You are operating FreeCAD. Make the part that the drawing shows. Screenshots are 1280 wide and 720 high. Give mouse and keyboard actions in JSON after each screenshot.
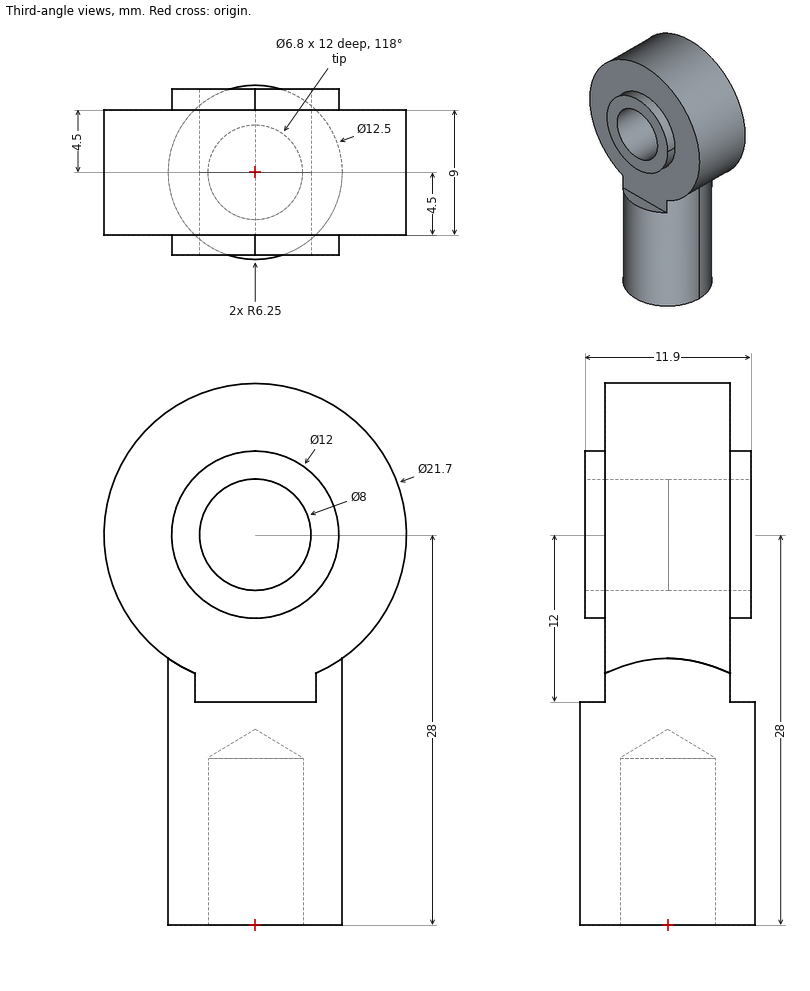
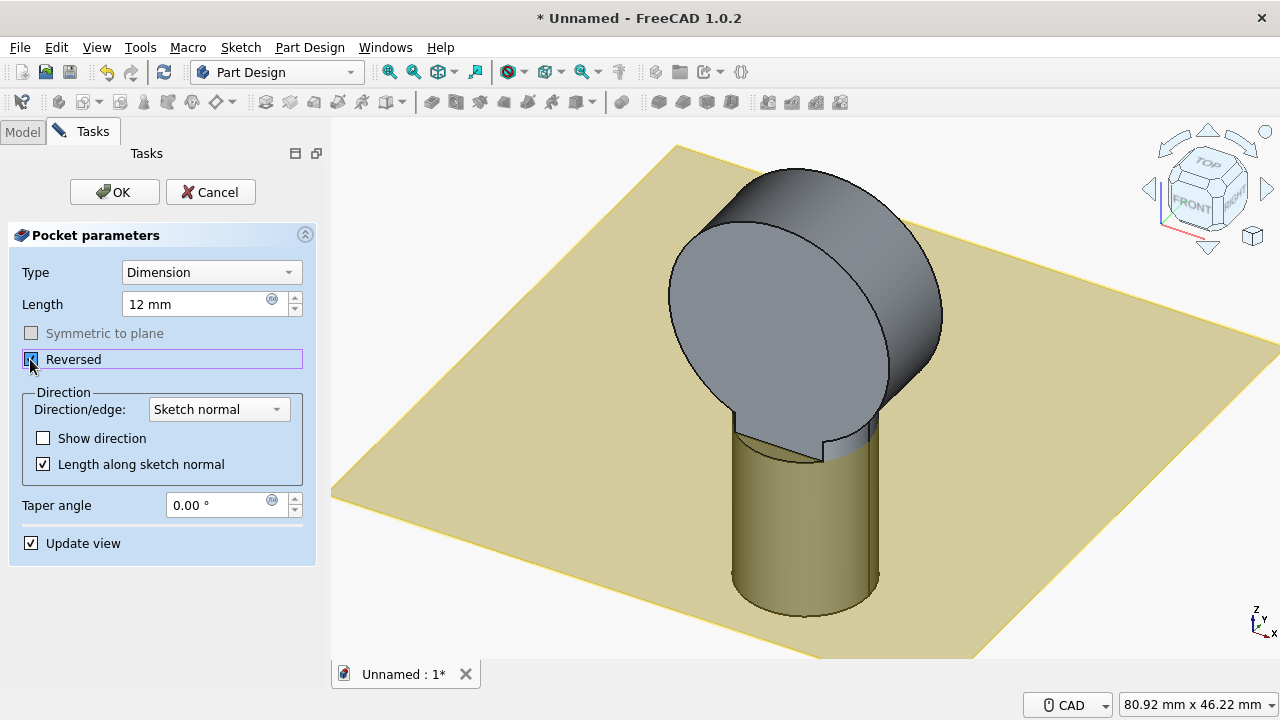
{"action": "left_click", "coordinate": [115, 192]}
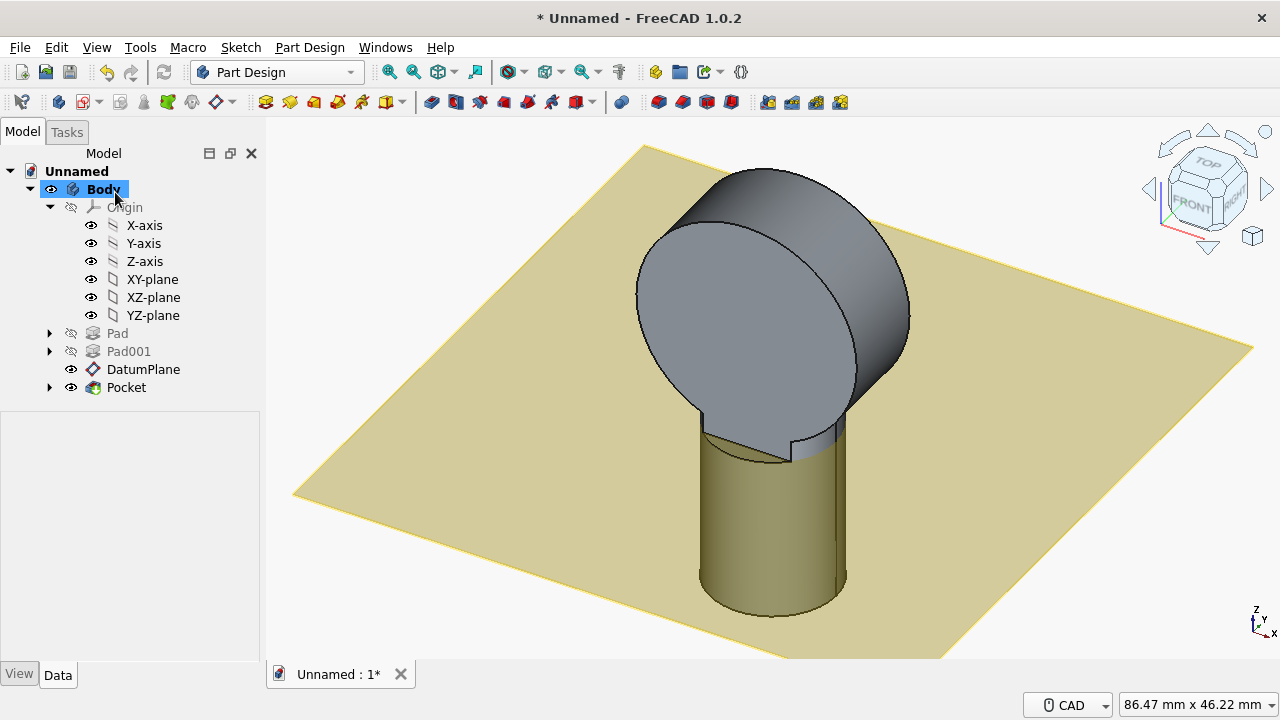
{"action": "left_click", "coordinate": [116, 369]}
{"action": "key", "text": "space"}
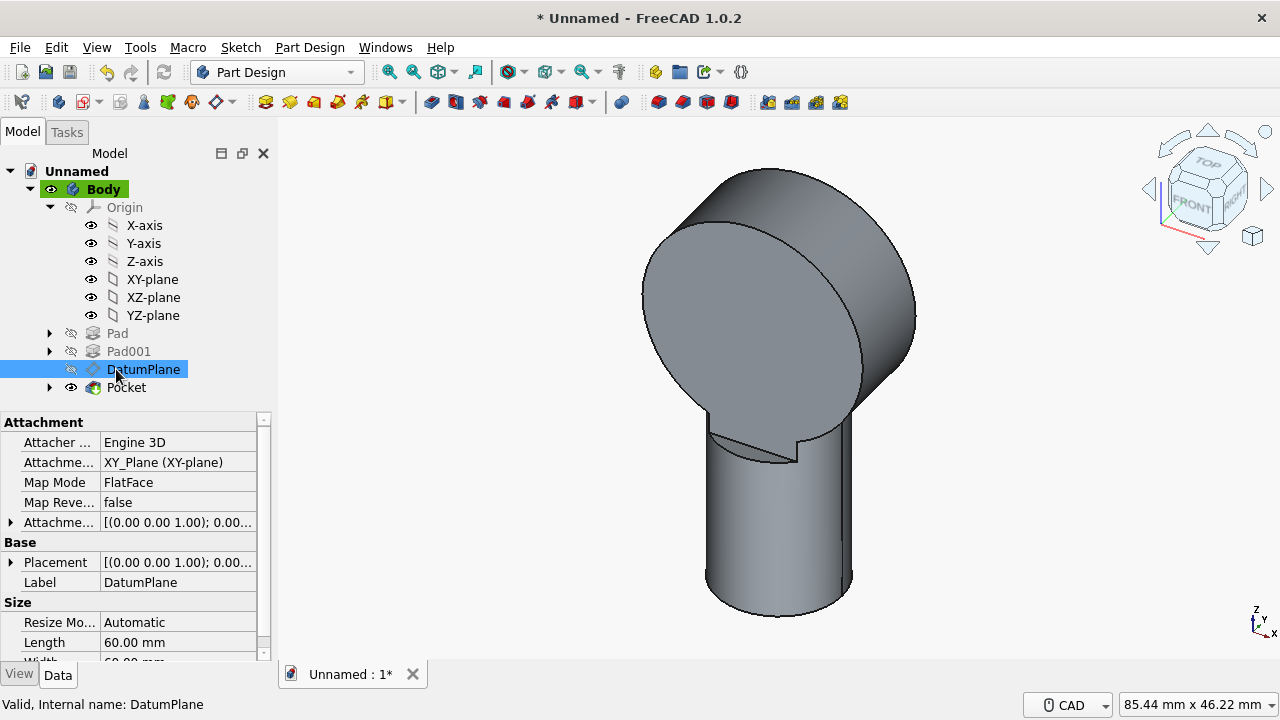
{"action": "left_click", "coordinate": [753, 336]}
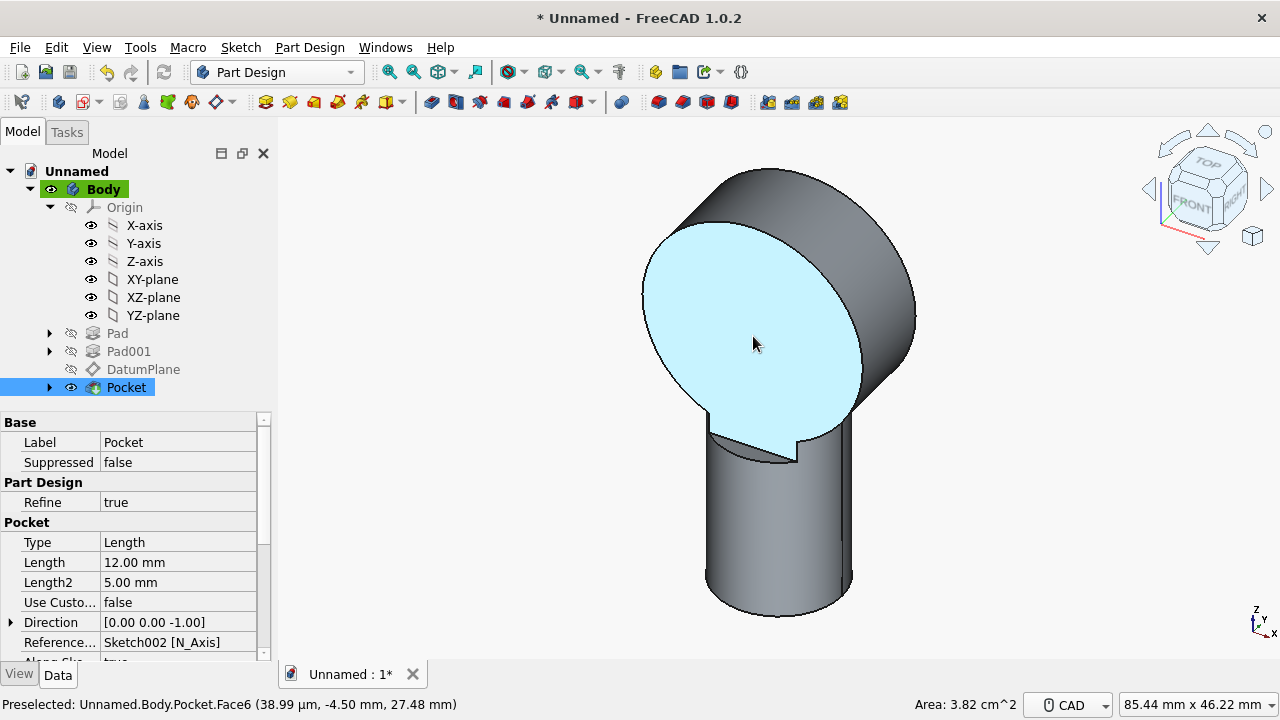
{"action": "left_click", "coordinate": [84, 102]}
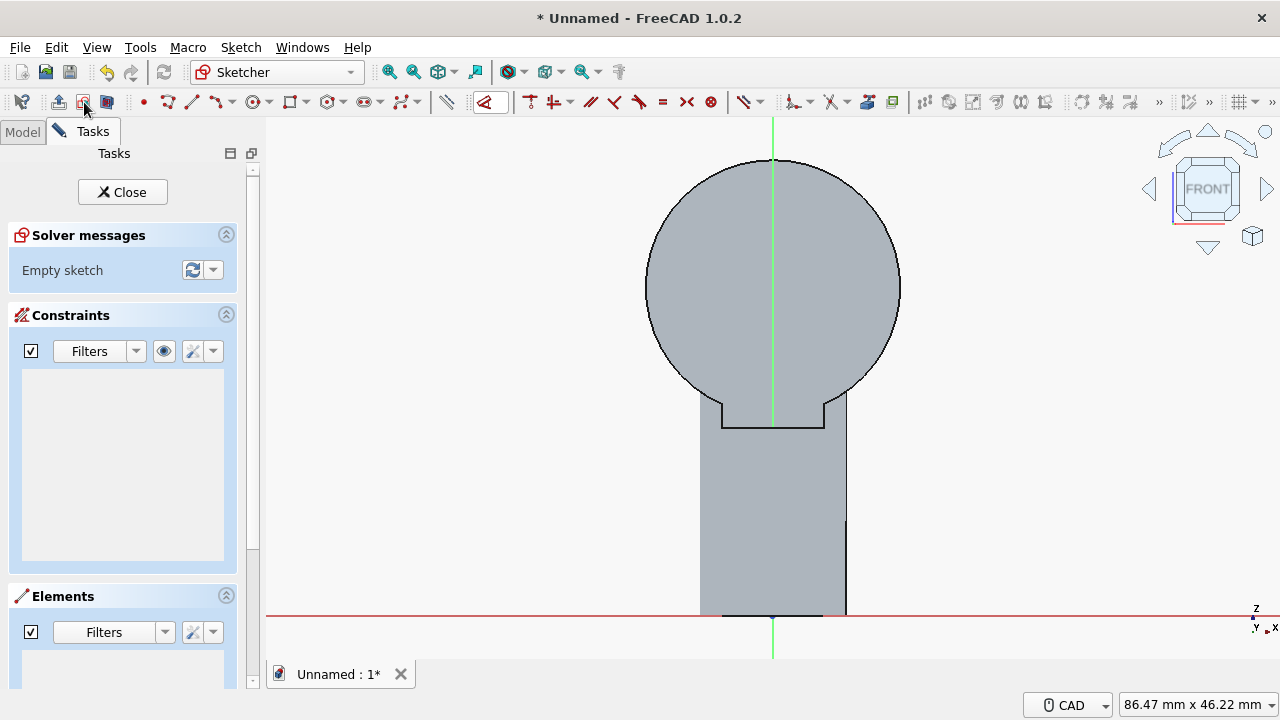
{"action": "key", "text": "q s"}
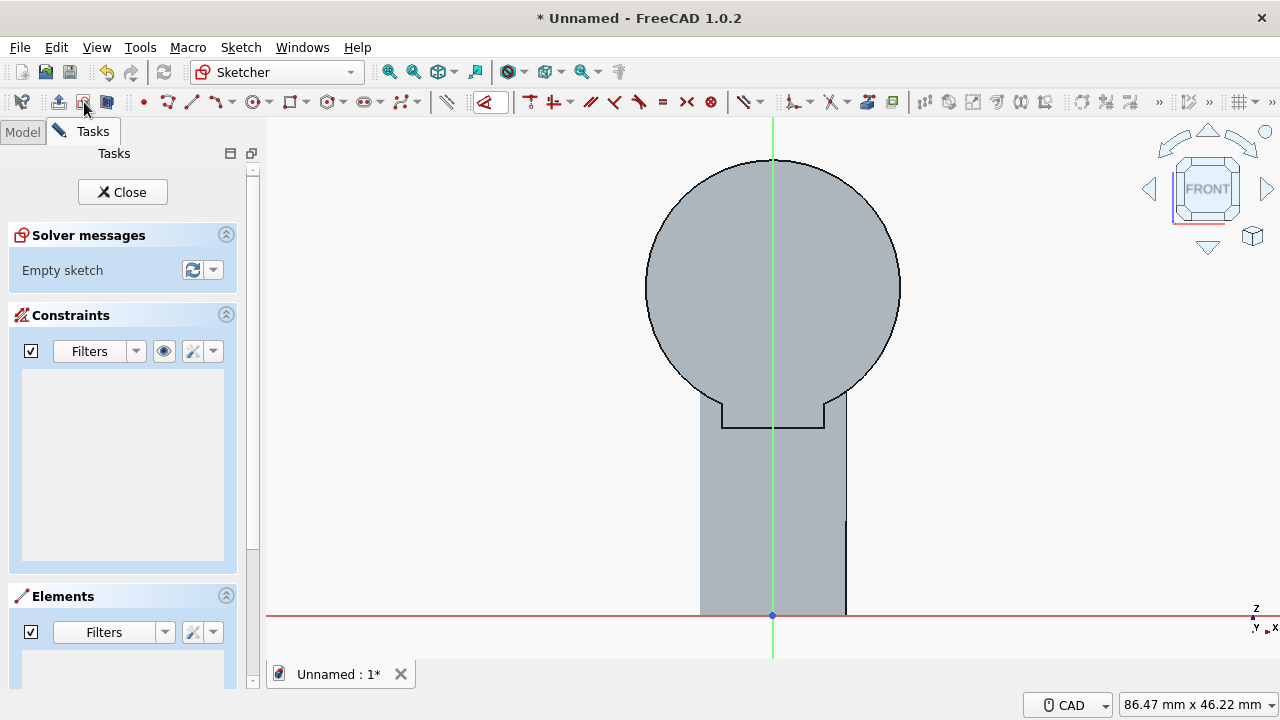
{"action": "scroll", "coordinate": [803, 244], "scroll_direction": "up", "scroll_amount": 6}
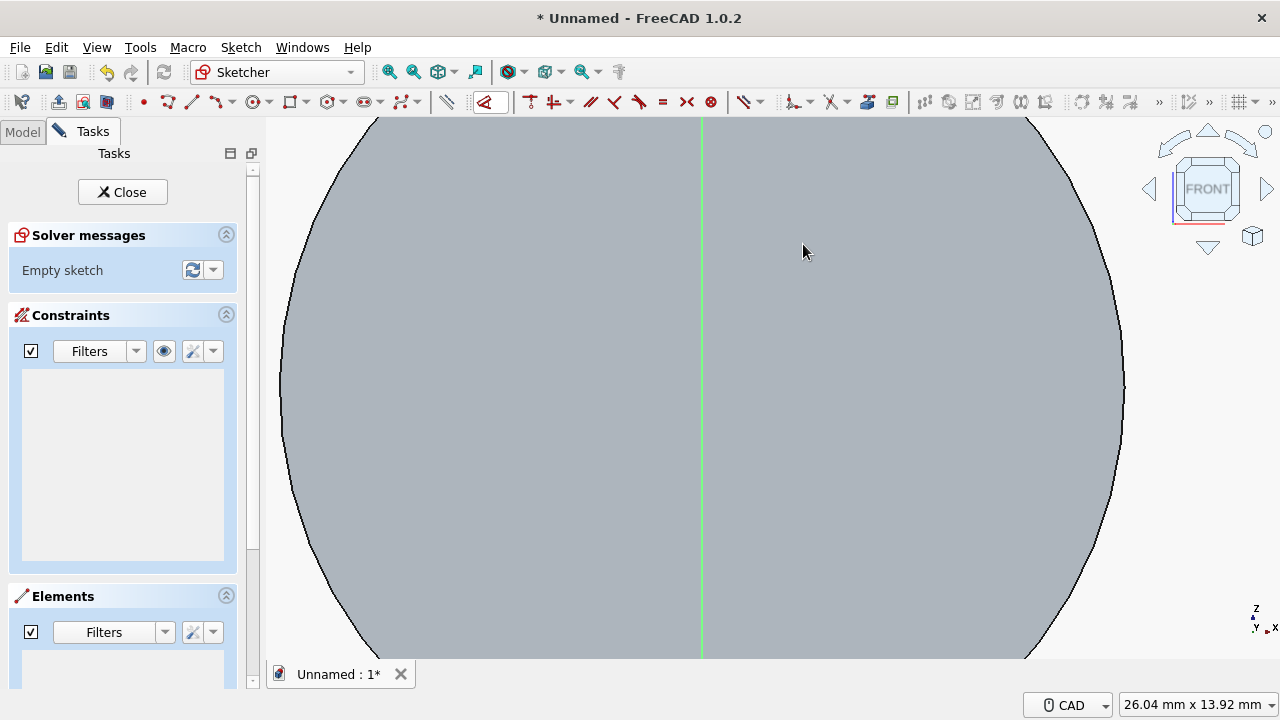
{"action": "left_click", "coordinate": [254, 102]}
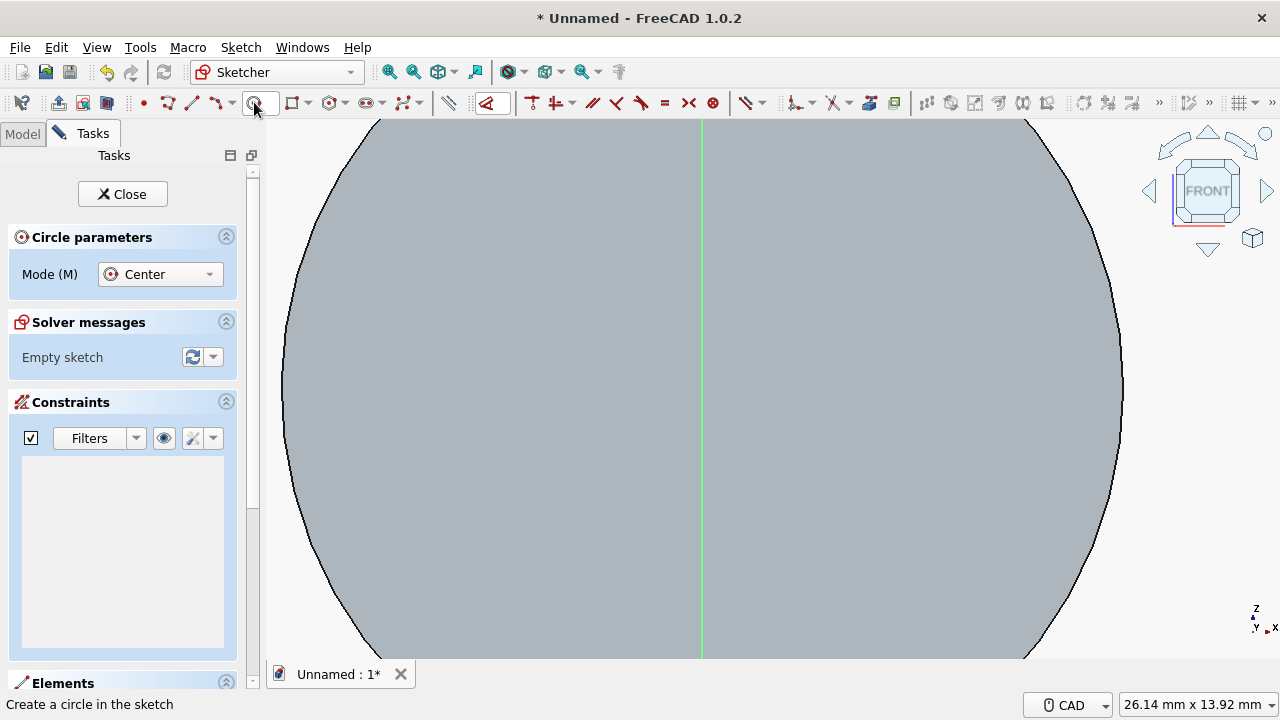
{"action": "left_click", "coordinate": [702, 389]}
{"action": "left_click", "coordinate": [812, 279]}
{"action": "key", "text": "Escape"}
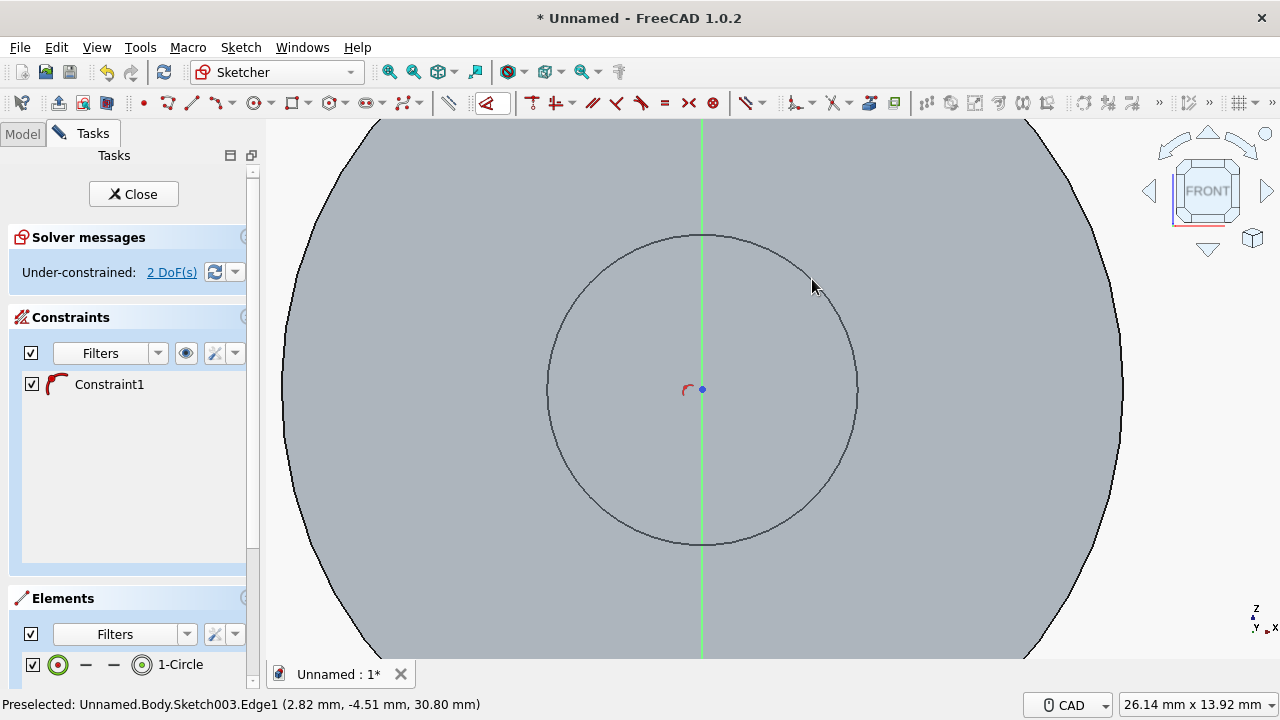
{"action": "left_click", "coordinate": [812, 280]}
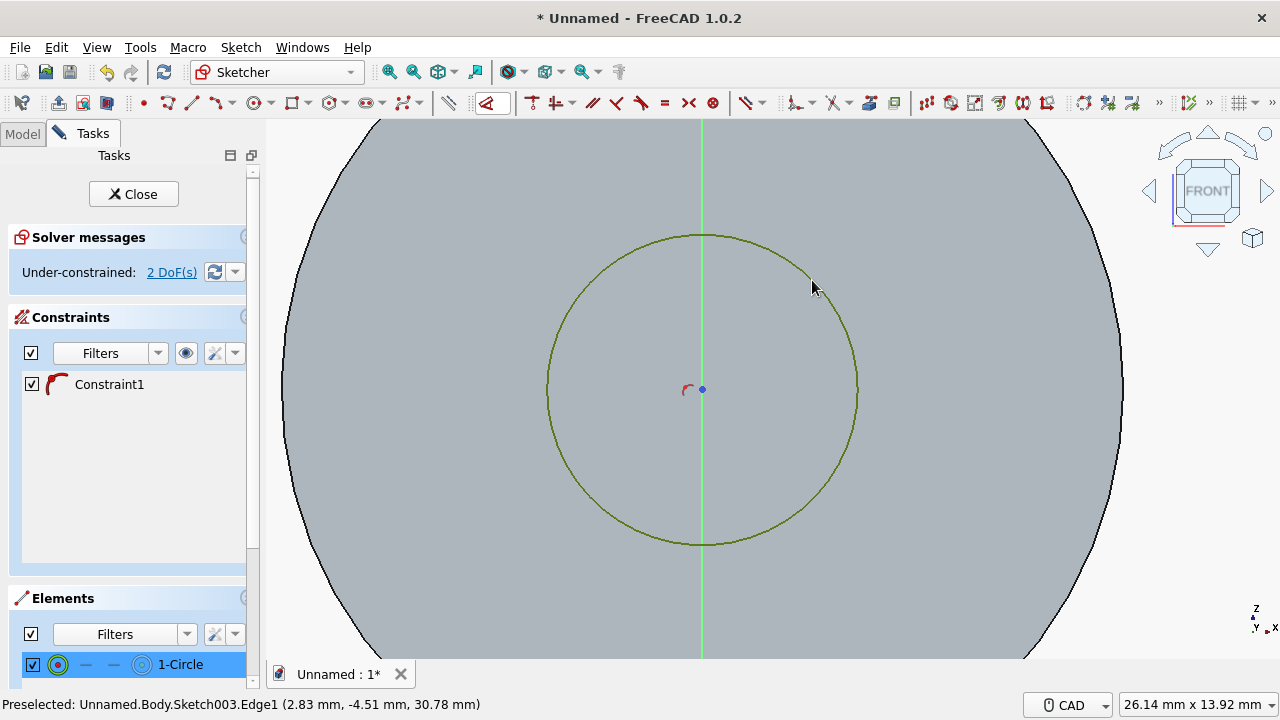
{"action": "left_click", "coordinate": [504, 104]}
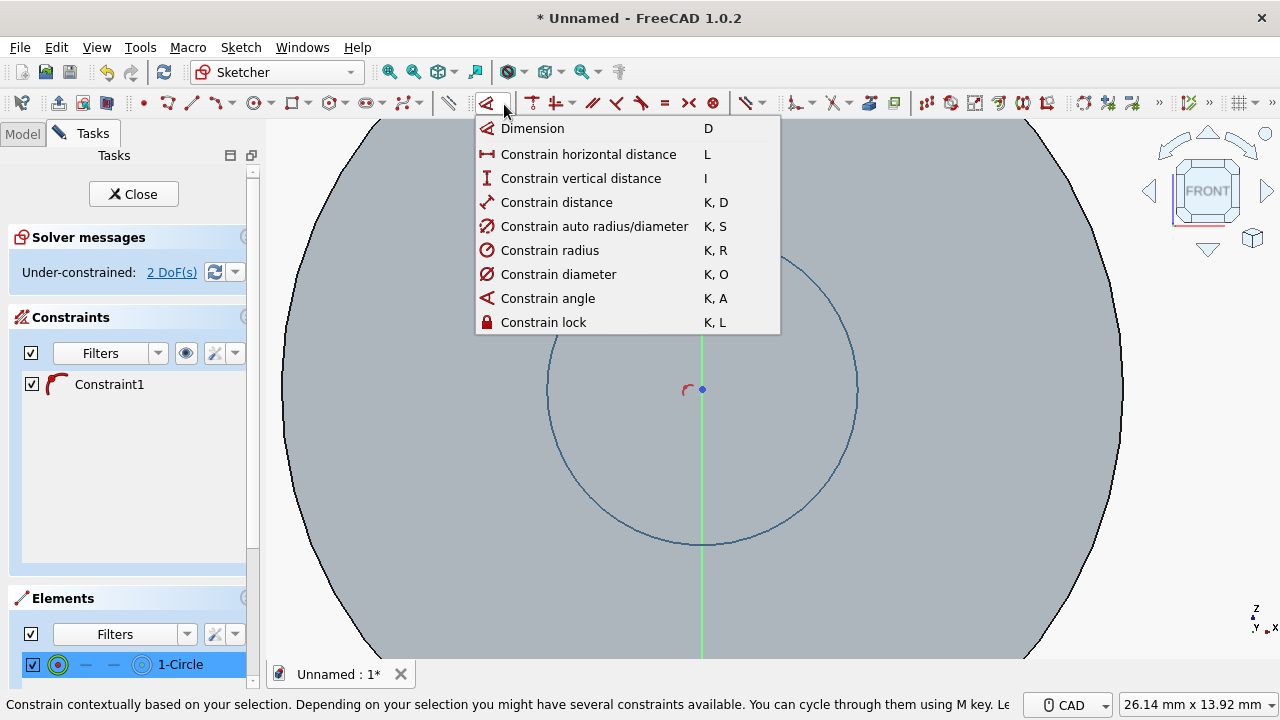
{"action": "left_click", "coordinate": [628, 274]}